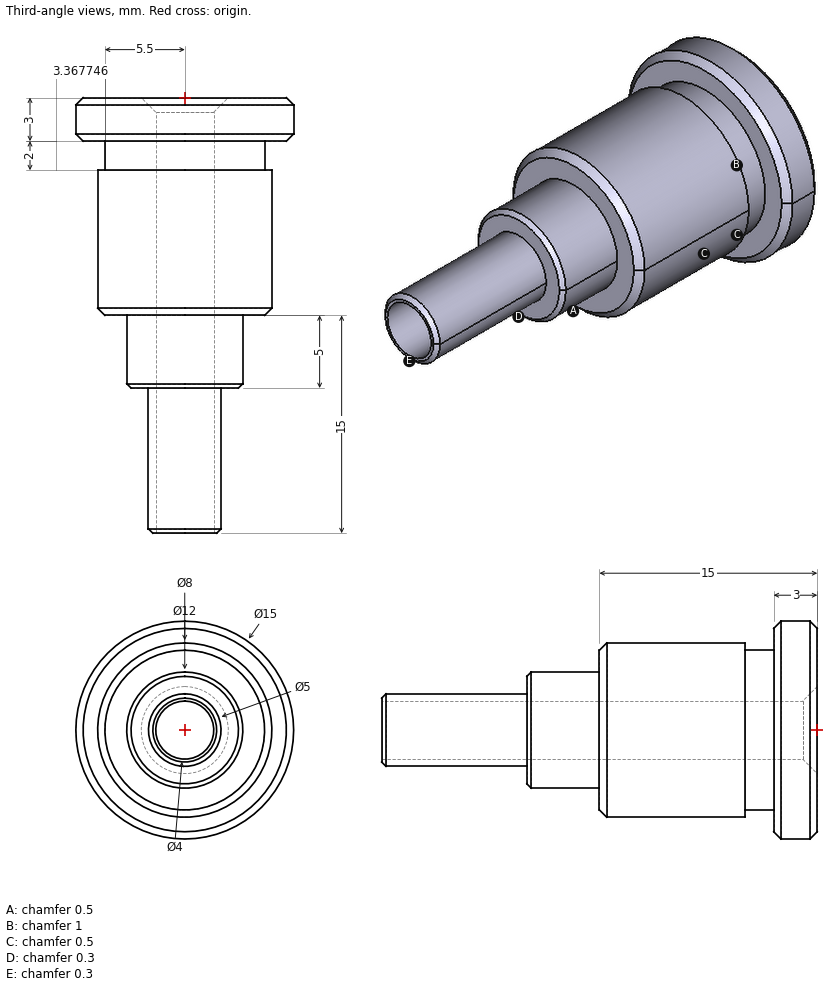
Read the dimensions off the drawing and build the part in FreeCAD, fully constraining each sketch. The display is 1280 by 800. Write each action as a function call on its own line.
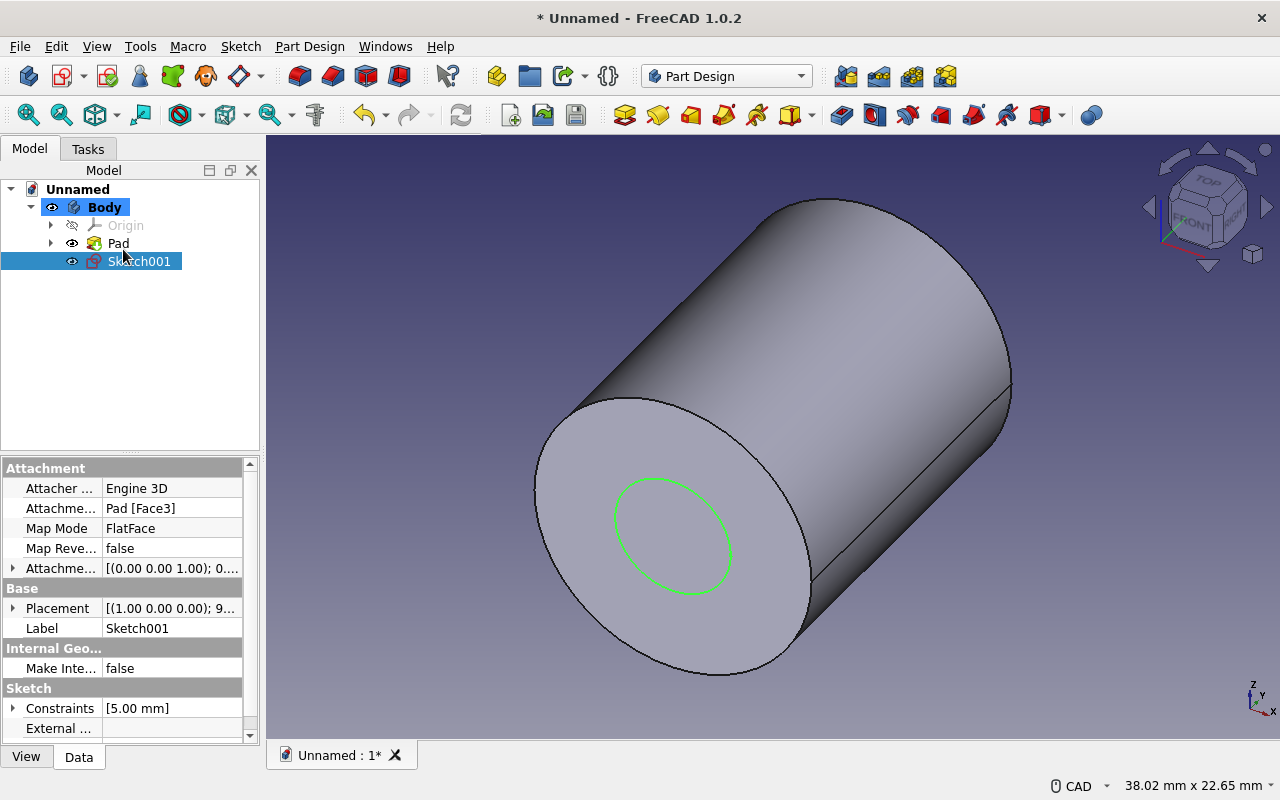
click(625, 116)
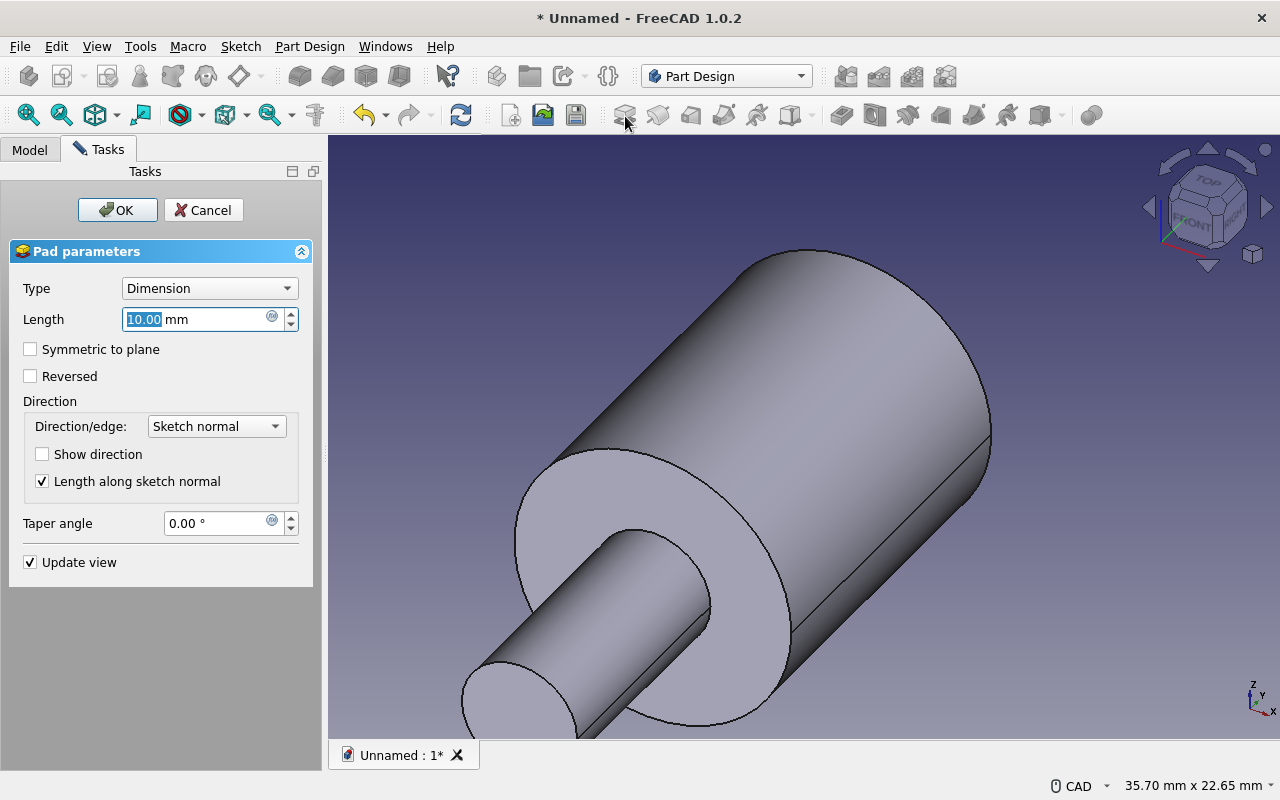
text(15)
key(Tab)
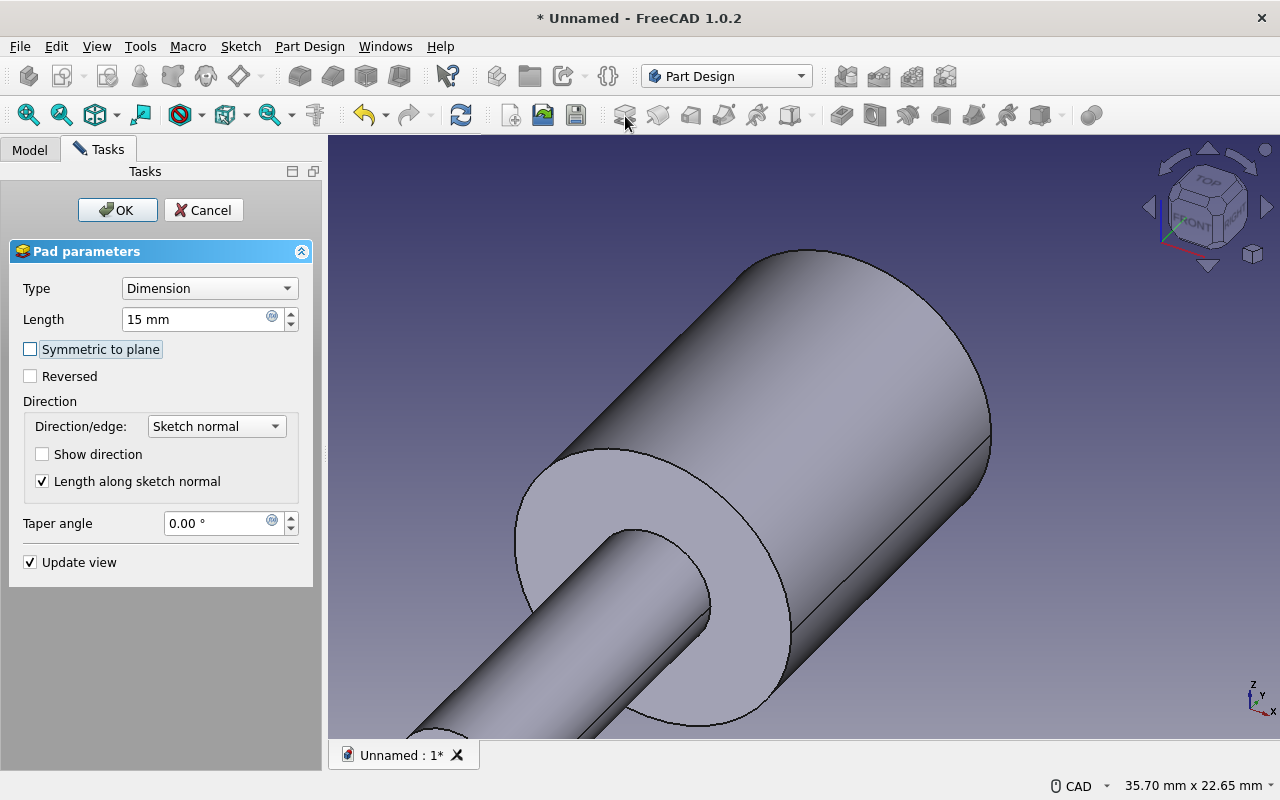
click(118, 210)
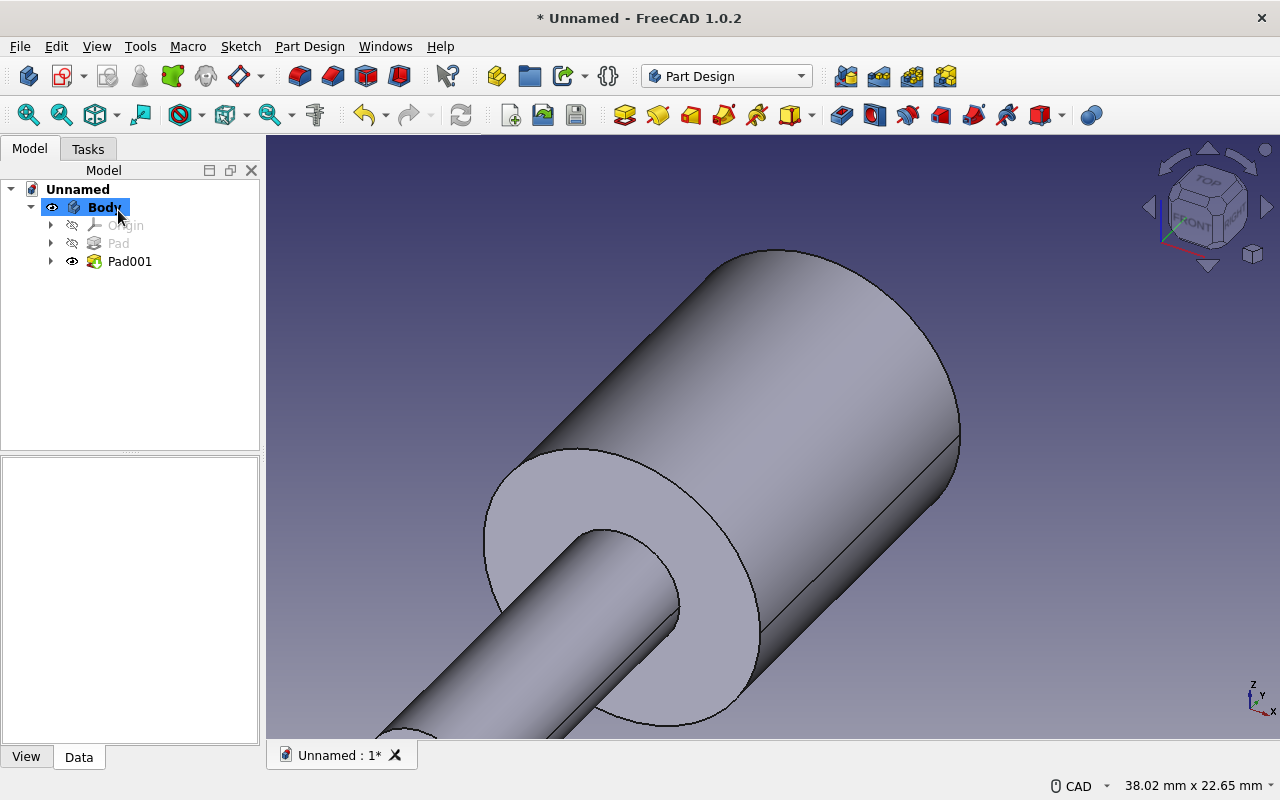
click(29, 116)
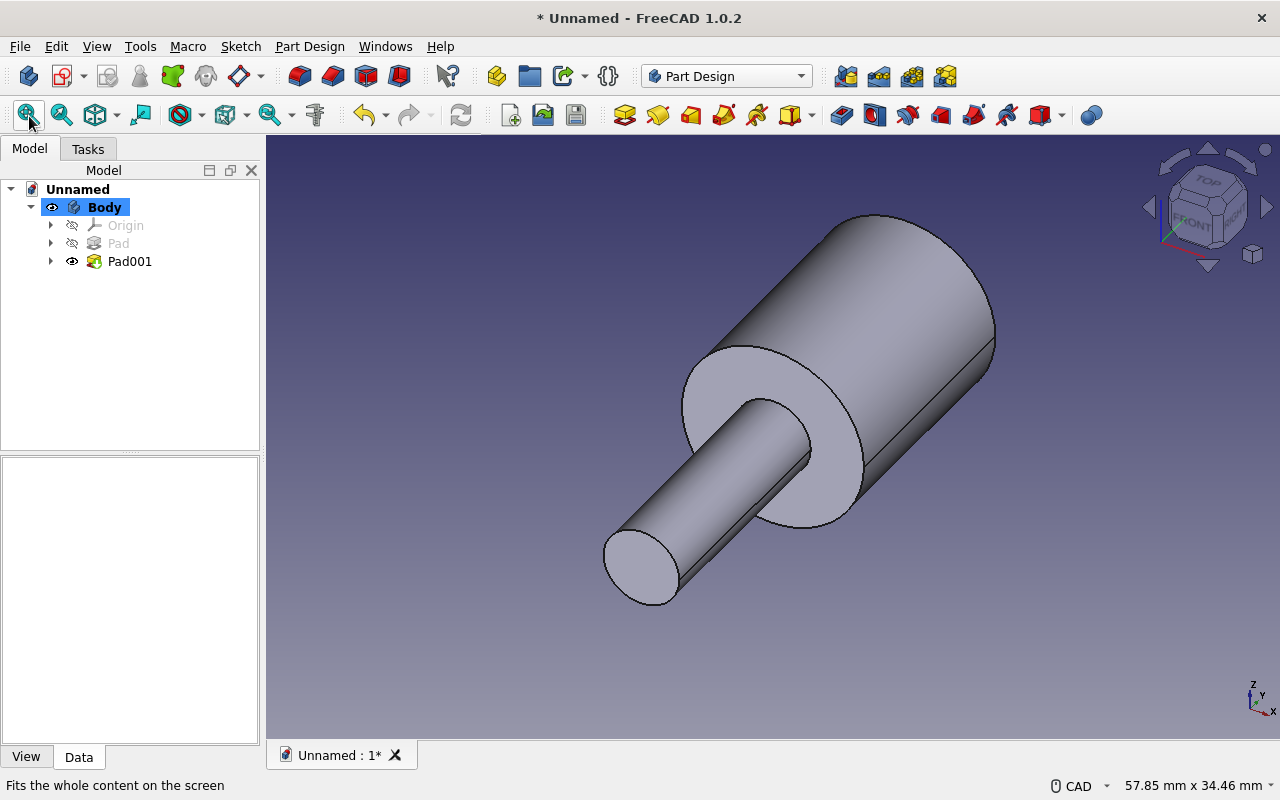
key(4)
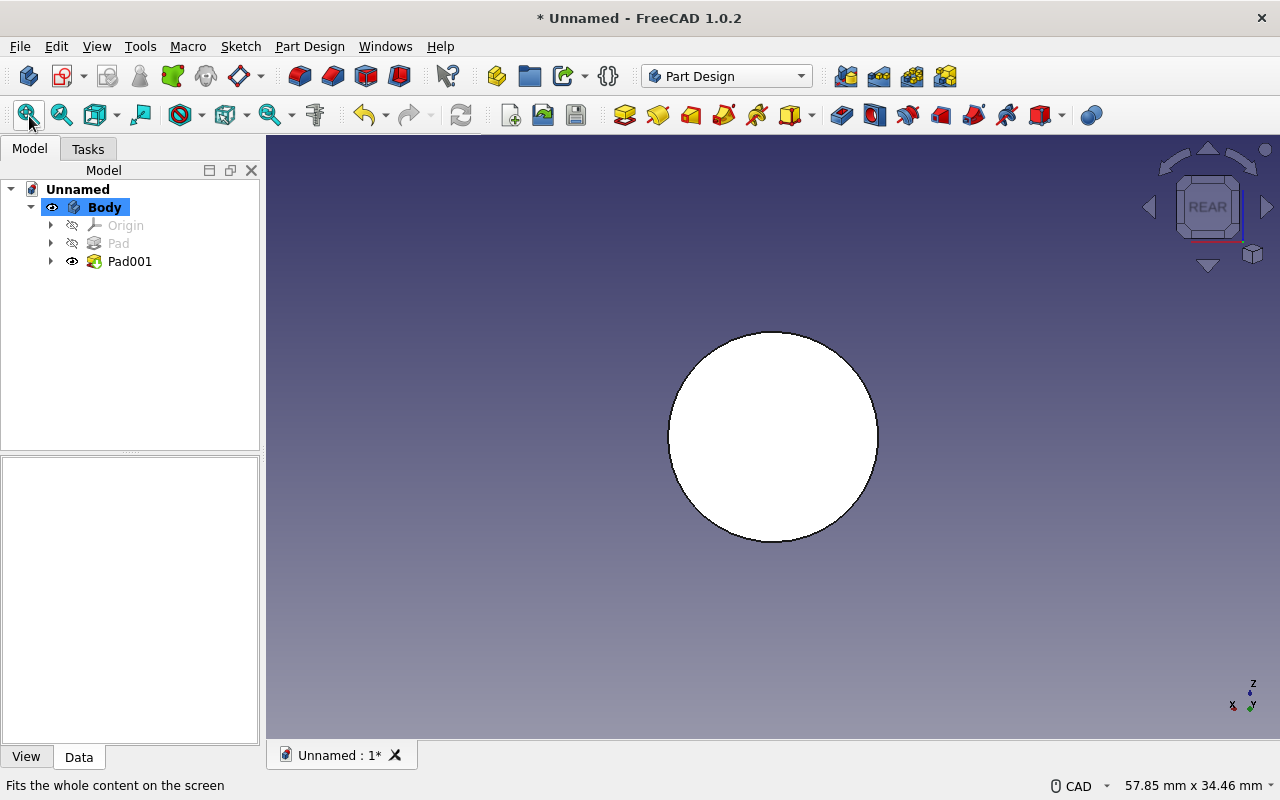
click(29, 116)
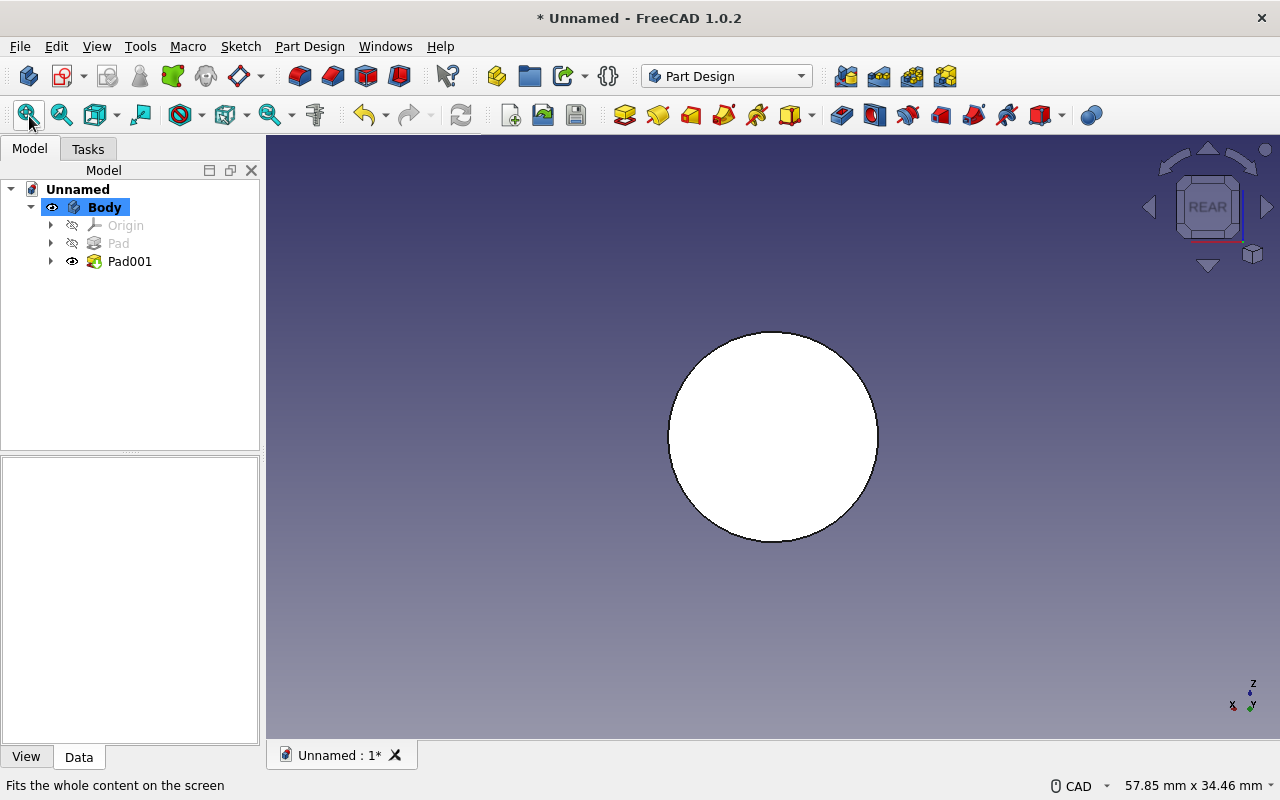
click(773, 436)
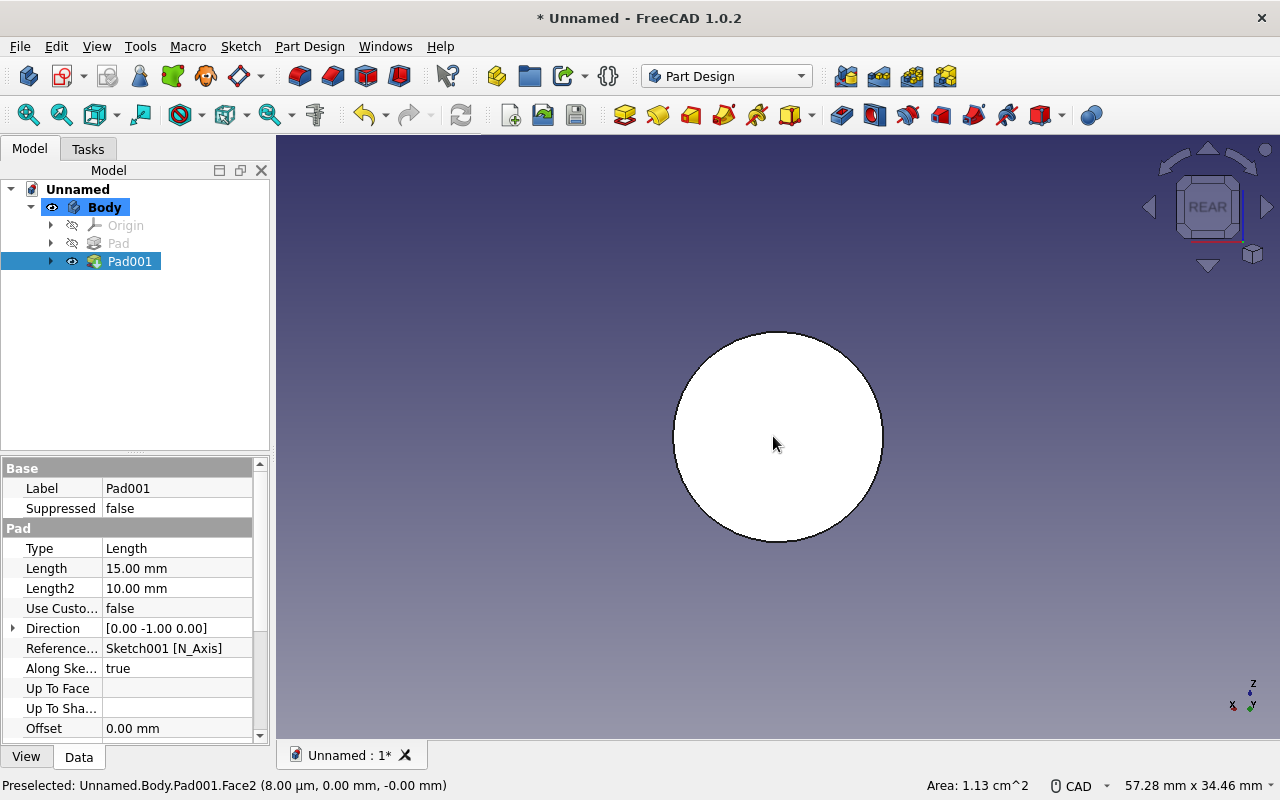
click(62, 76)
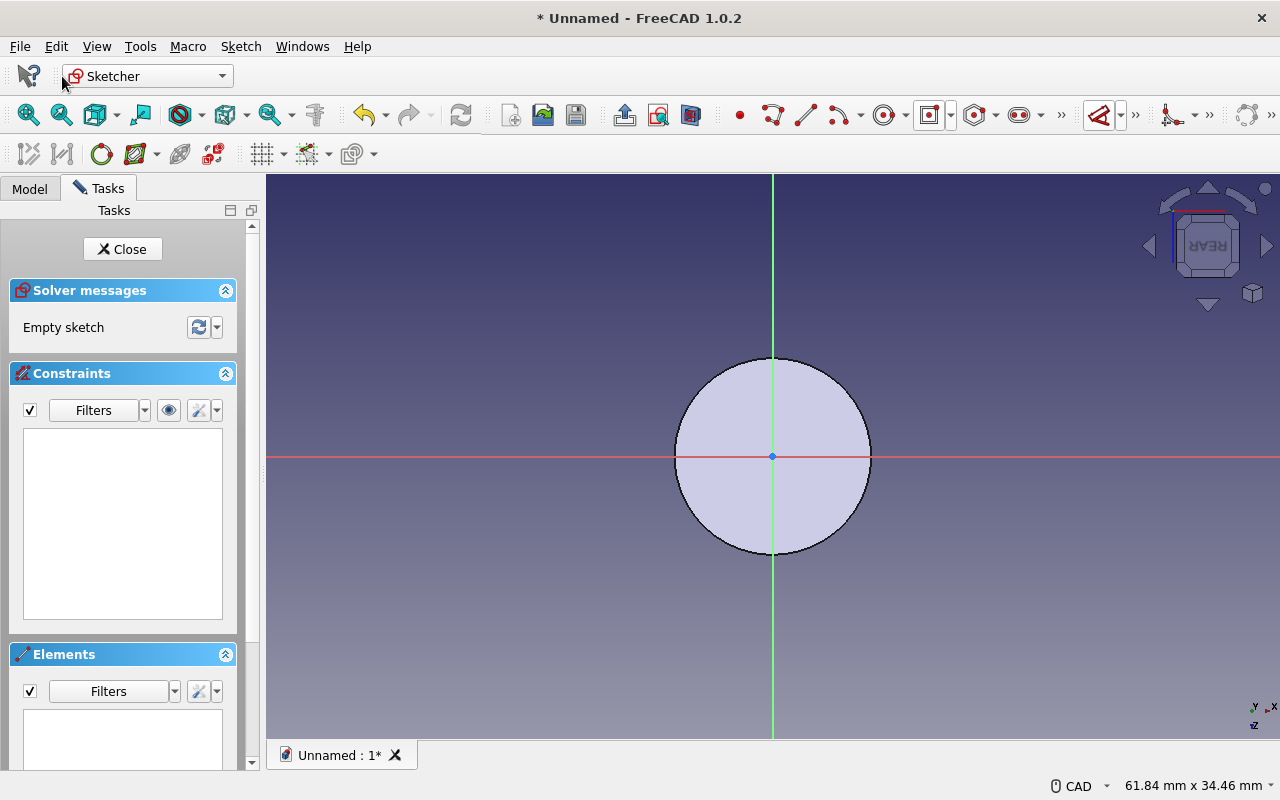
scroll(786, 457, up, 9)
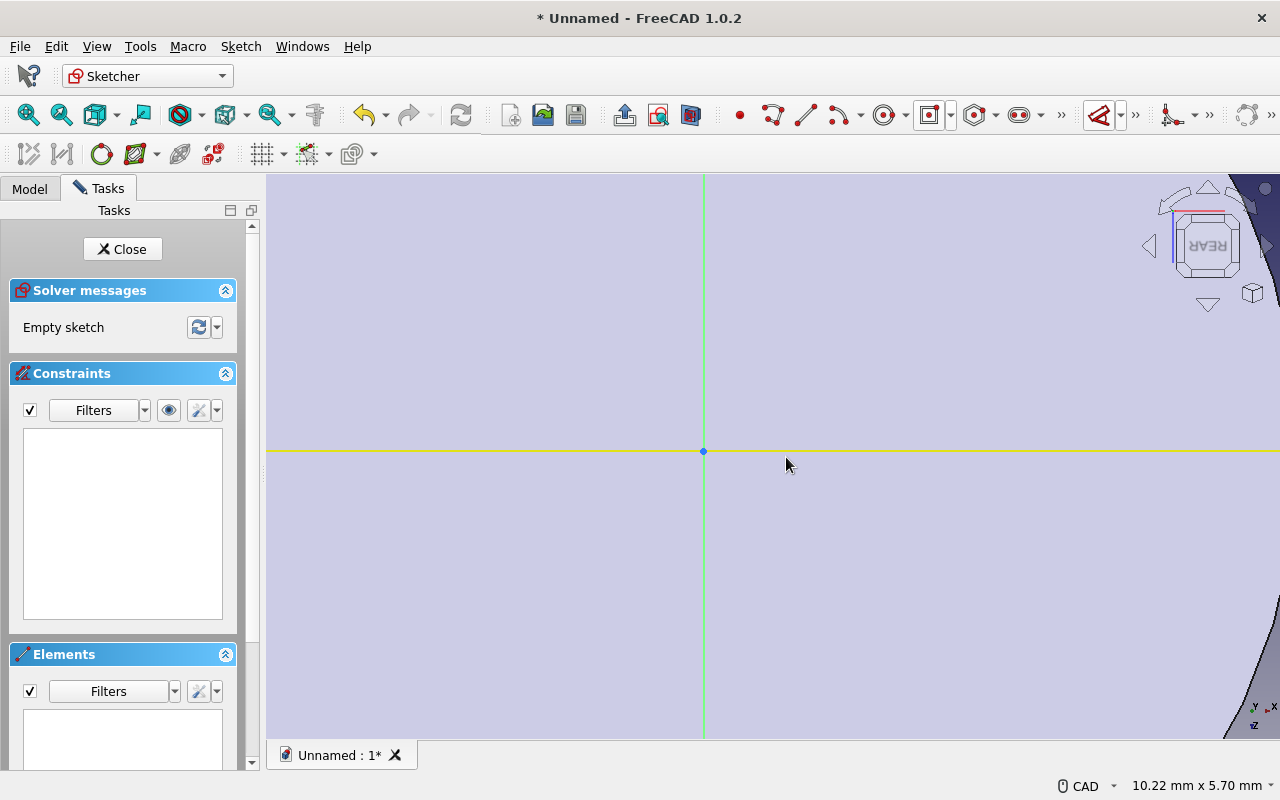
click(884, 116)